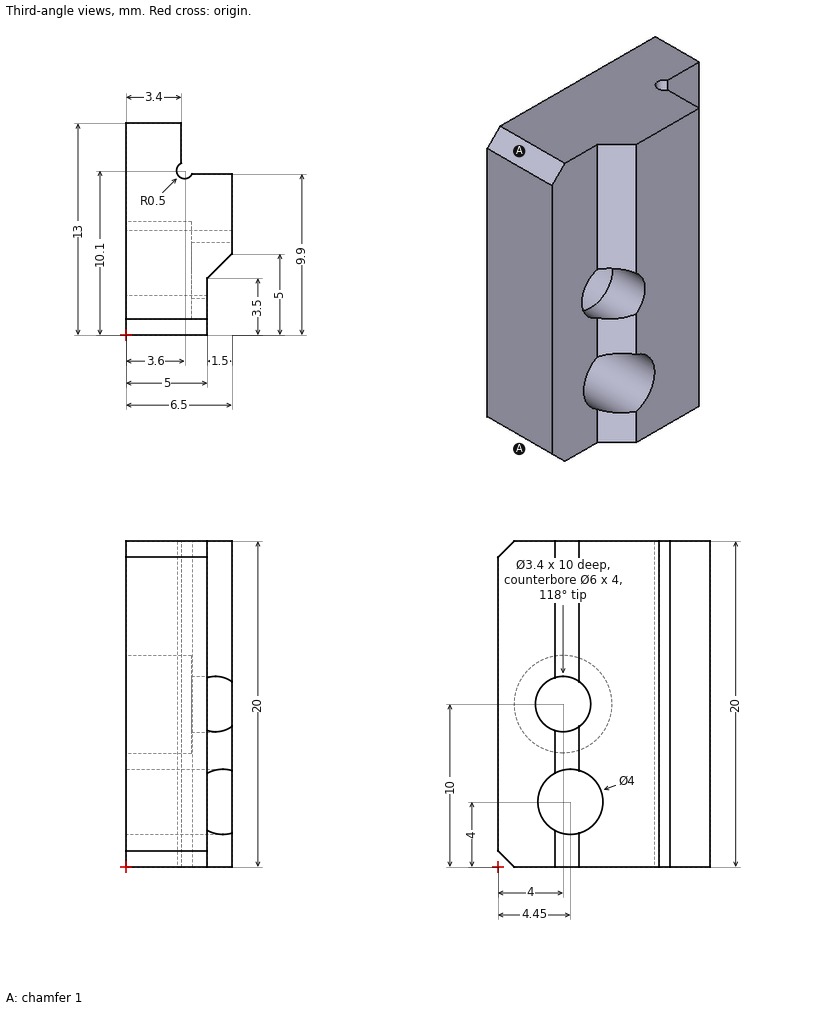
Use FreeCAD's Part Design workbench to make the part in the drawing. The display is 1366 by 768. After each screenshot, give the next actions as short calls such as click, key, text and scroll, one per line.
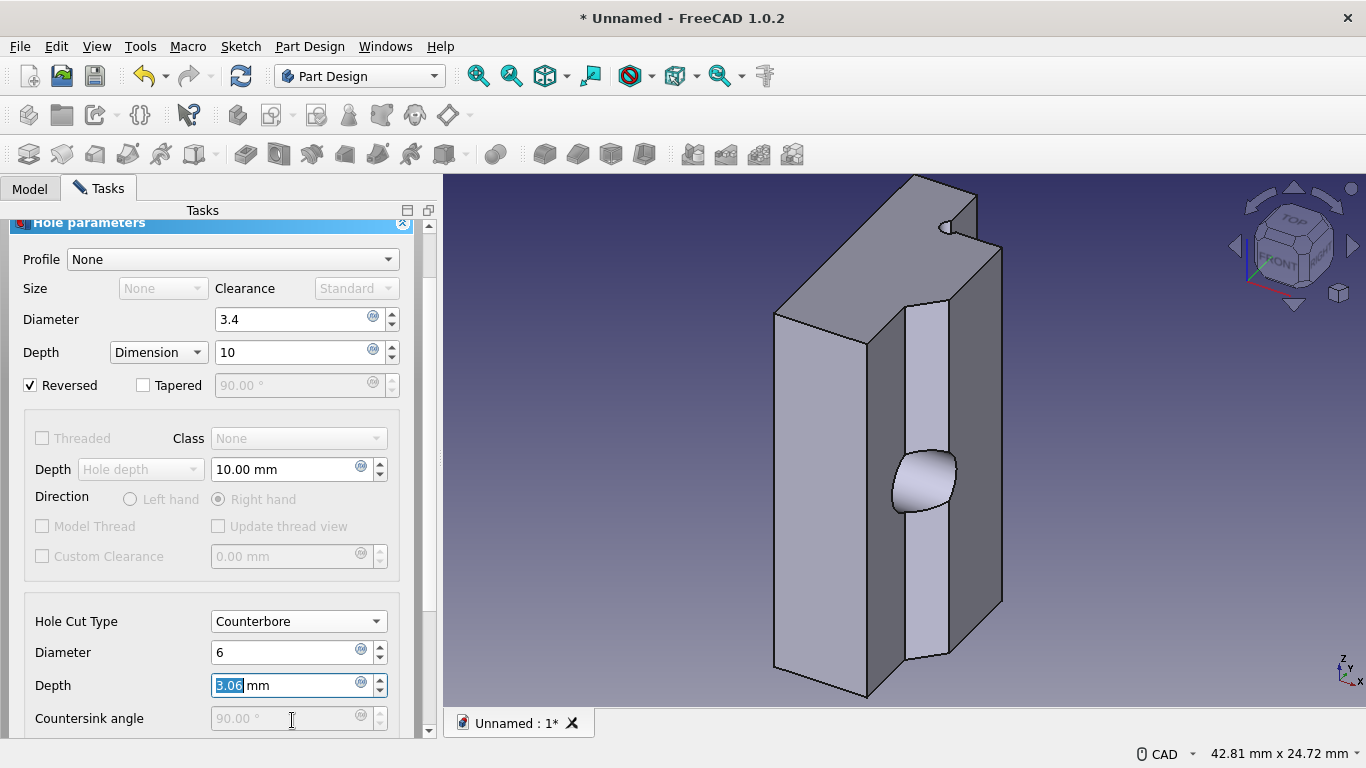
text(4)
key(Tab)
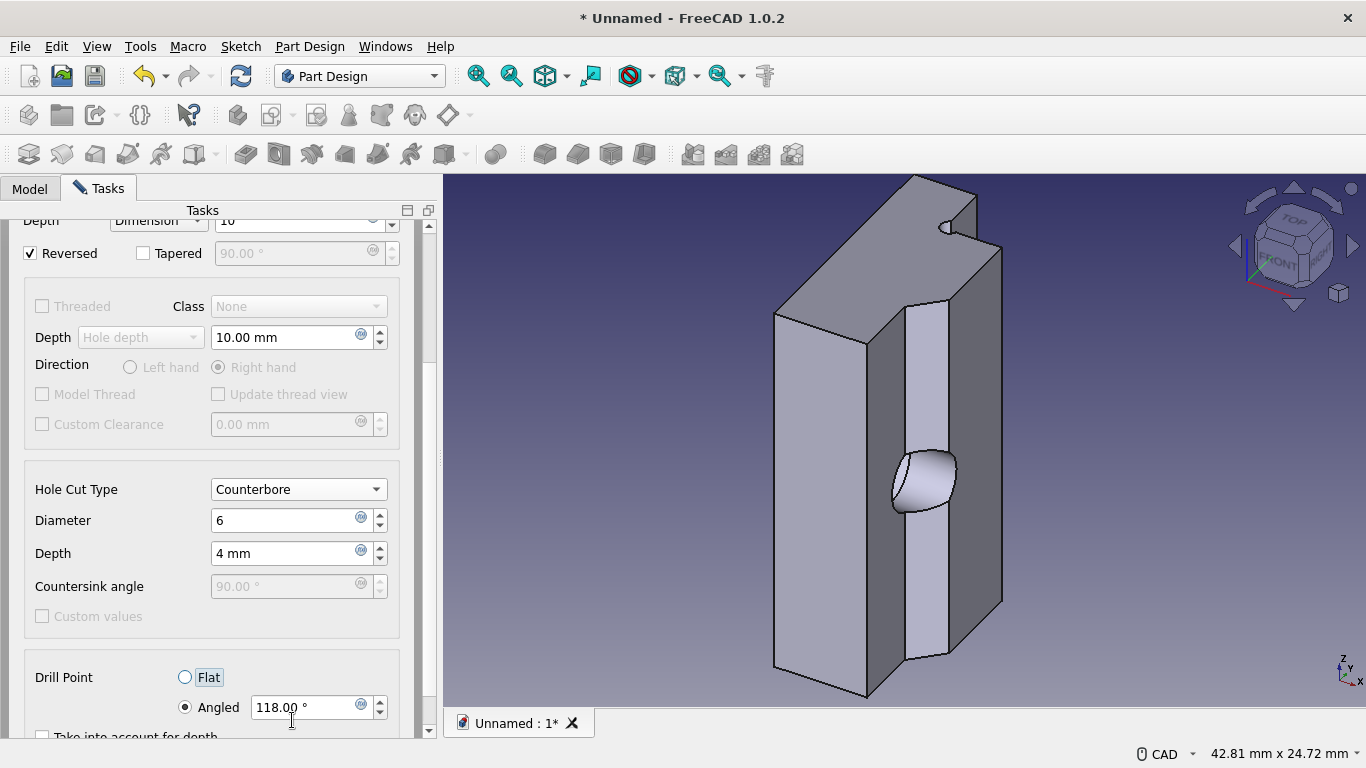
scroll(429, 479, up, 5)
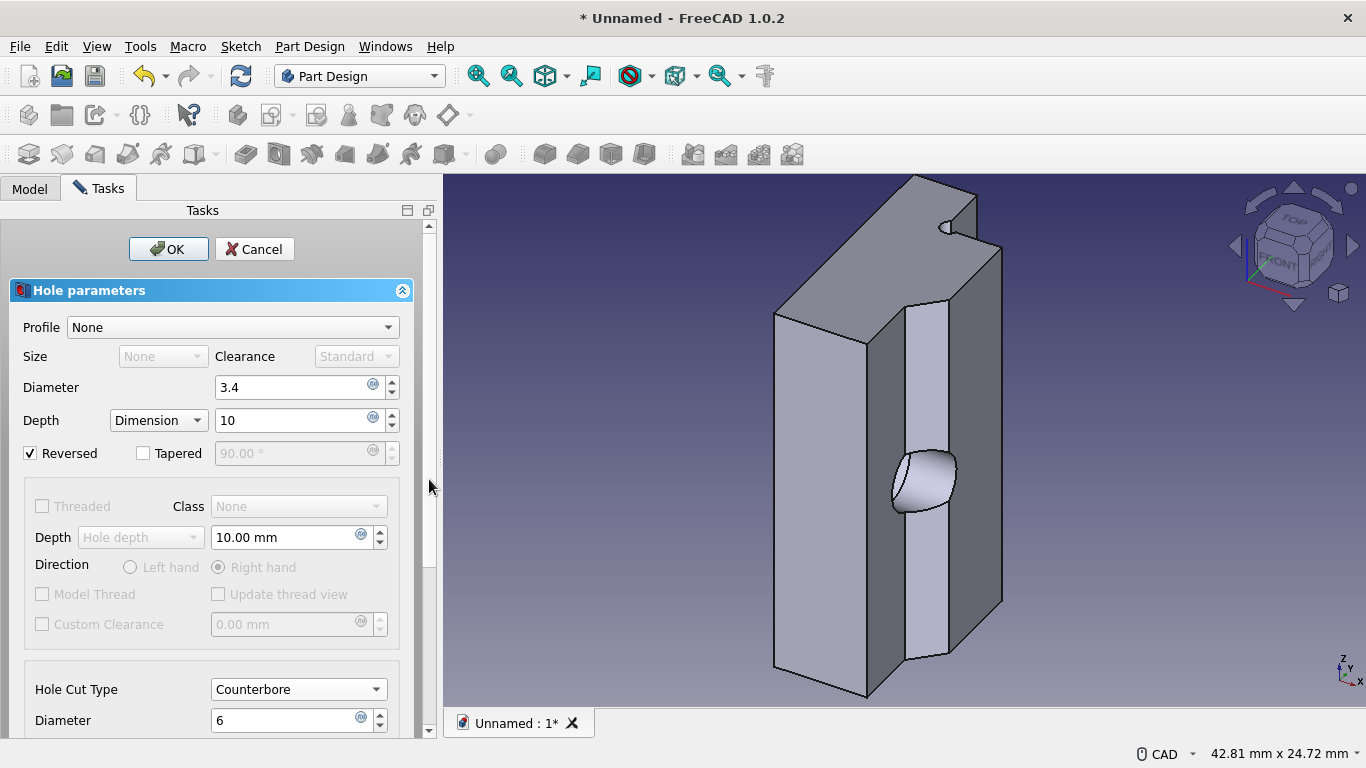
click(169, 249)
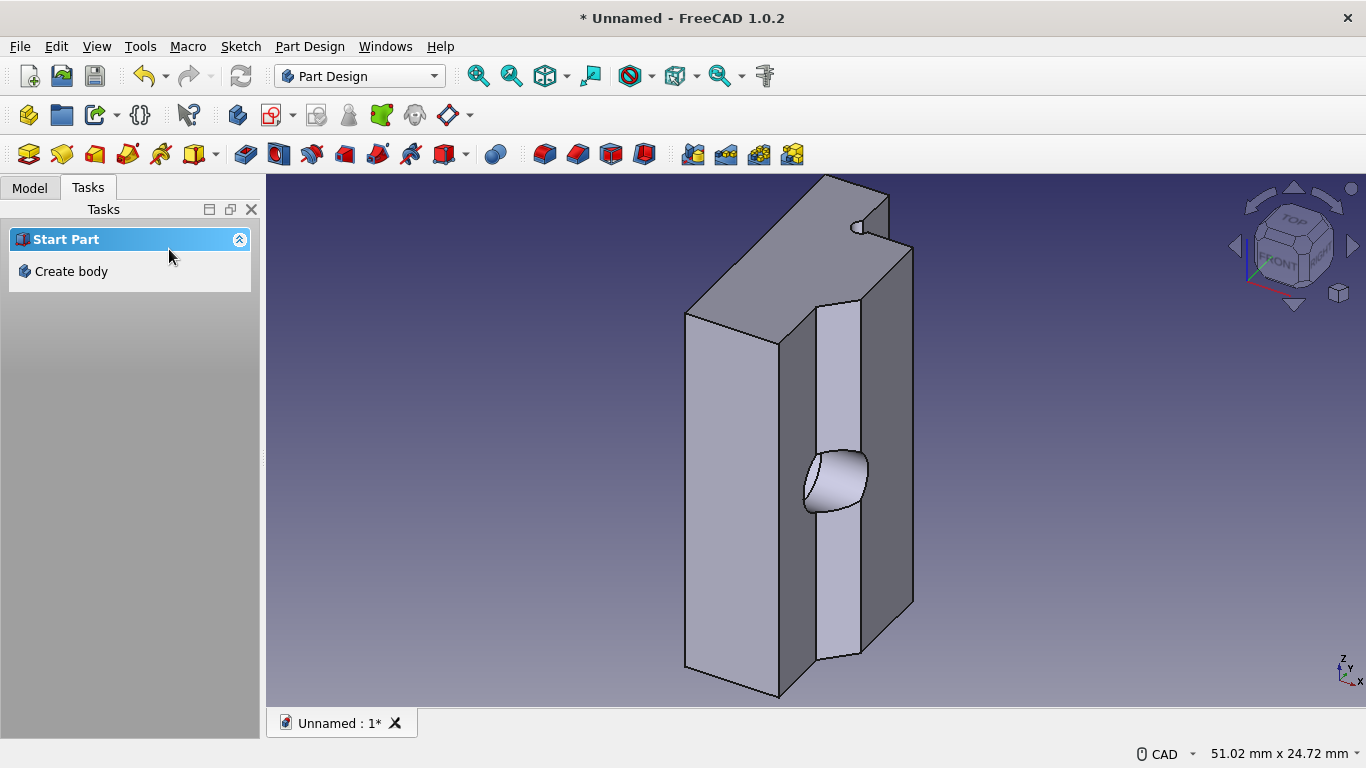
click(479, 76)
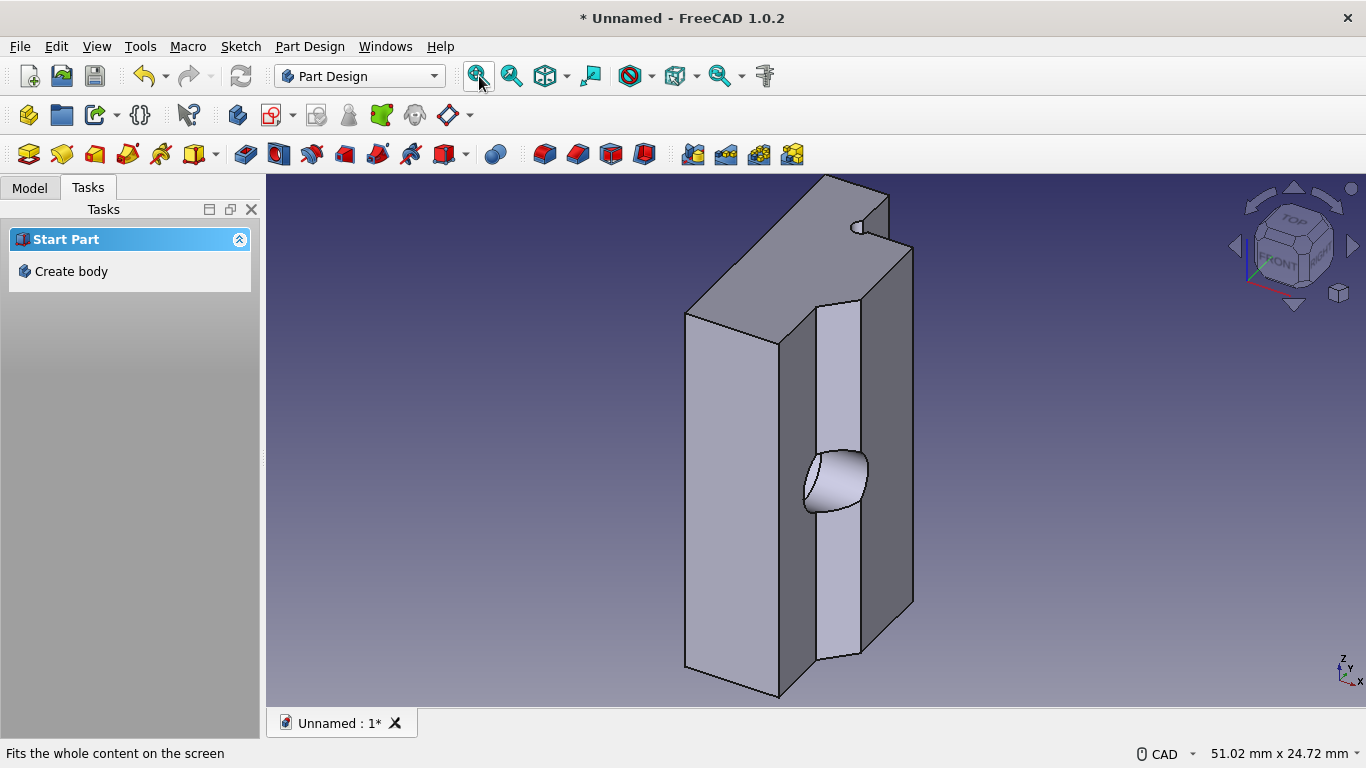
click(732, 328)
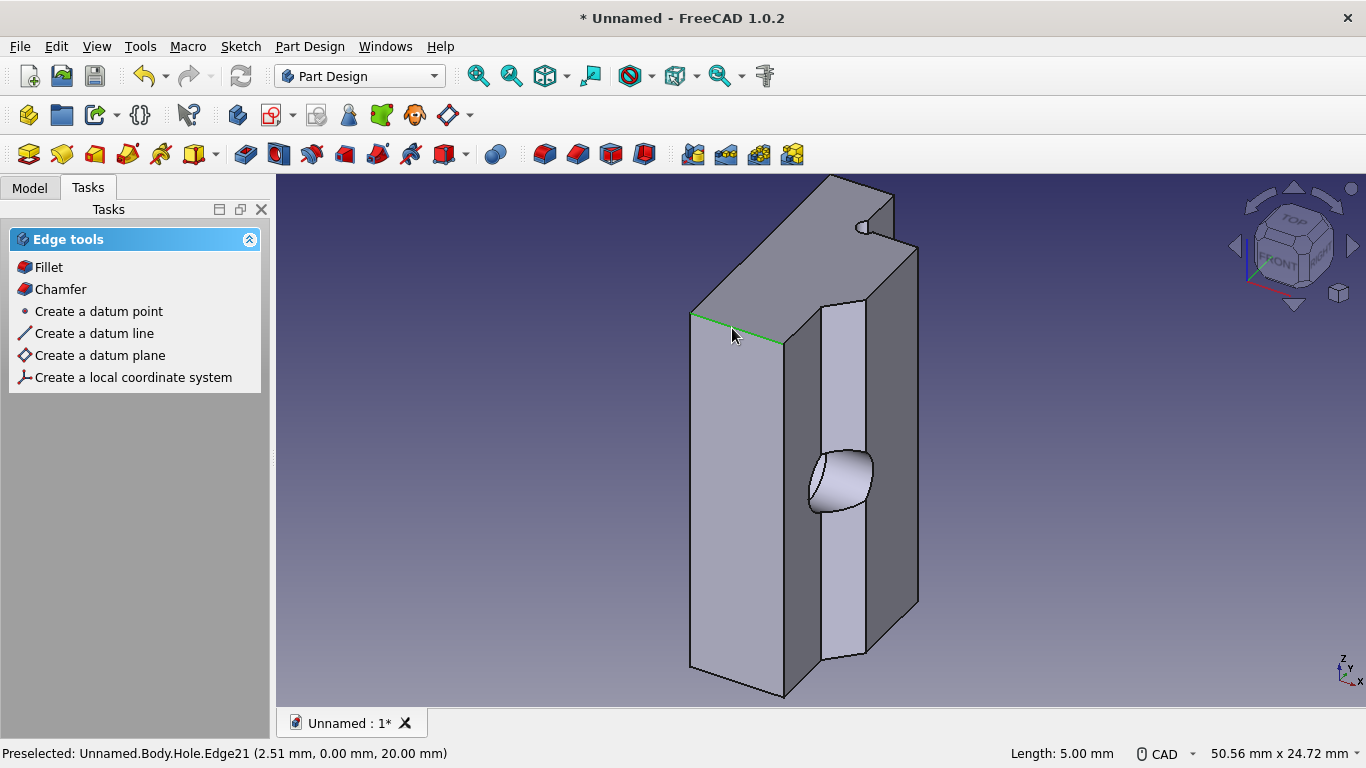
key(0)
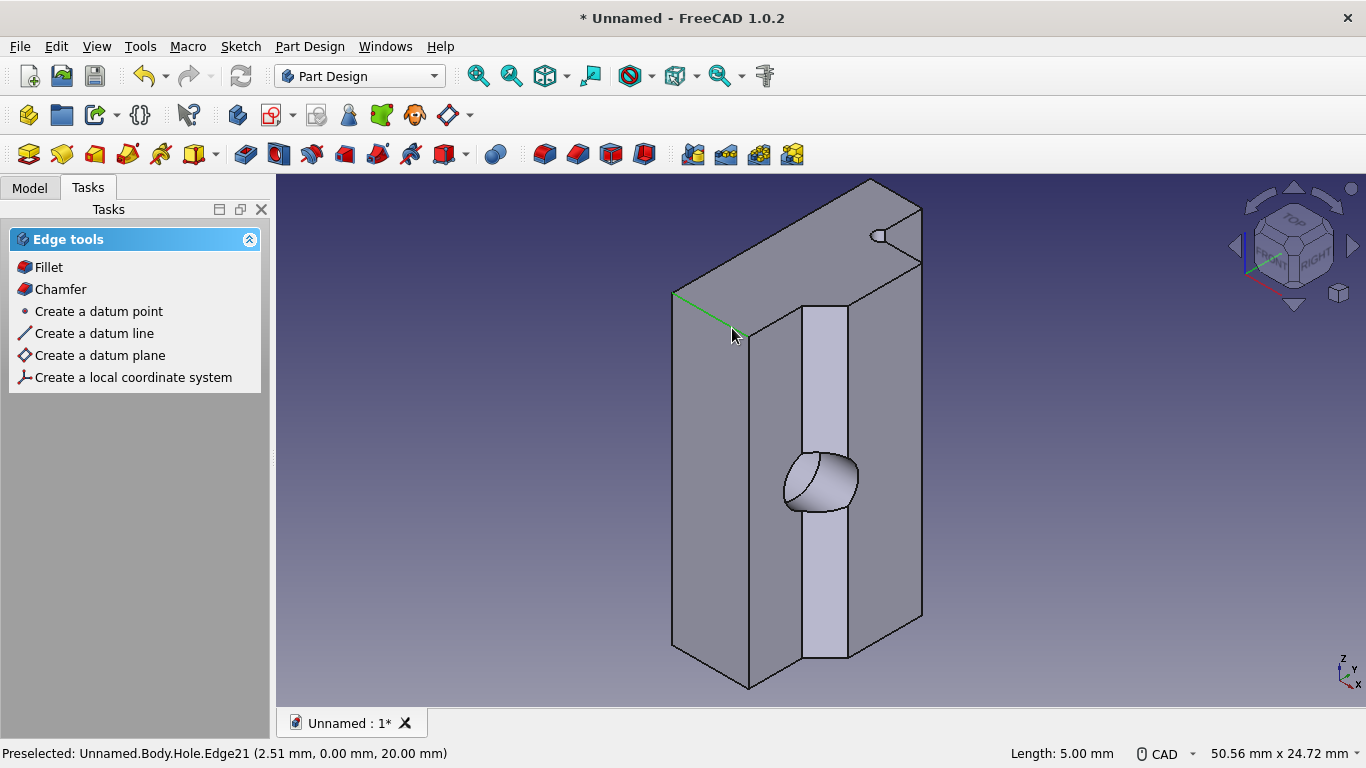
key(2)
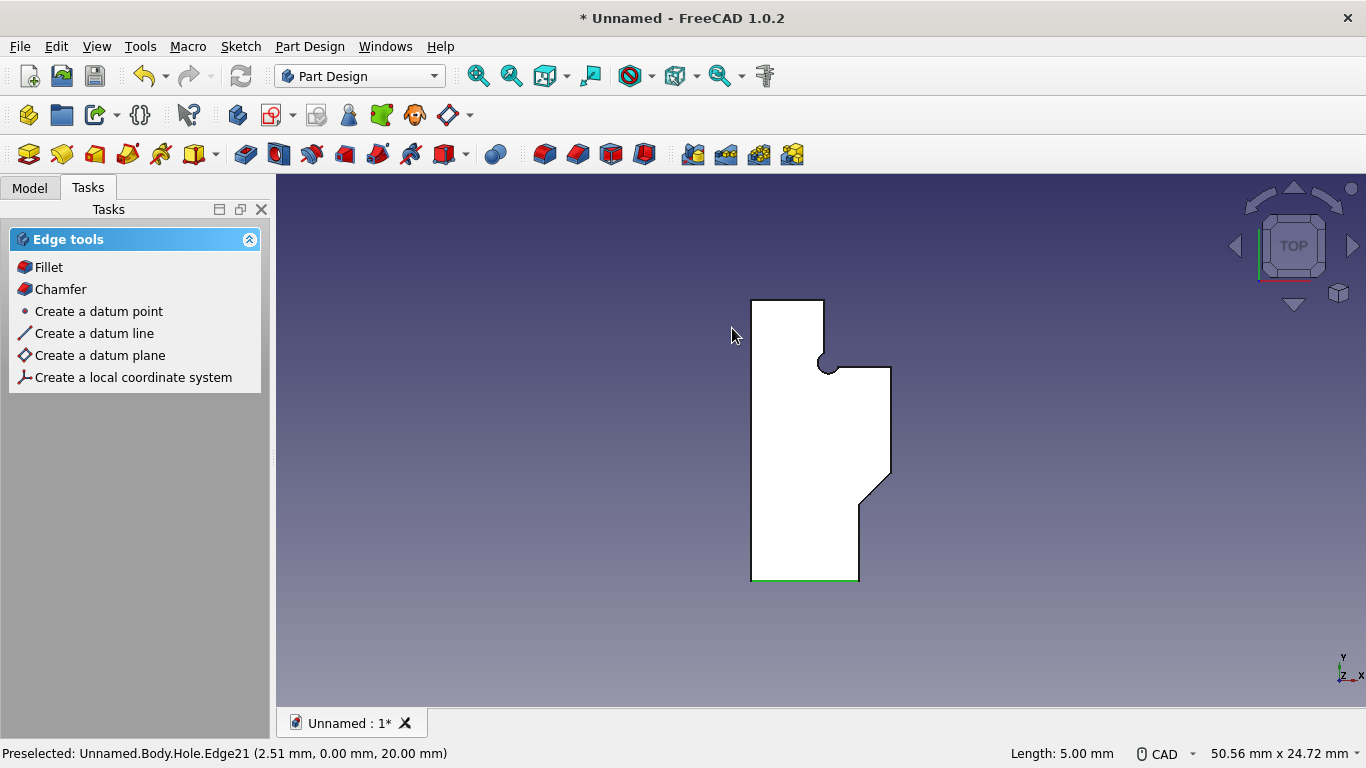
key(1)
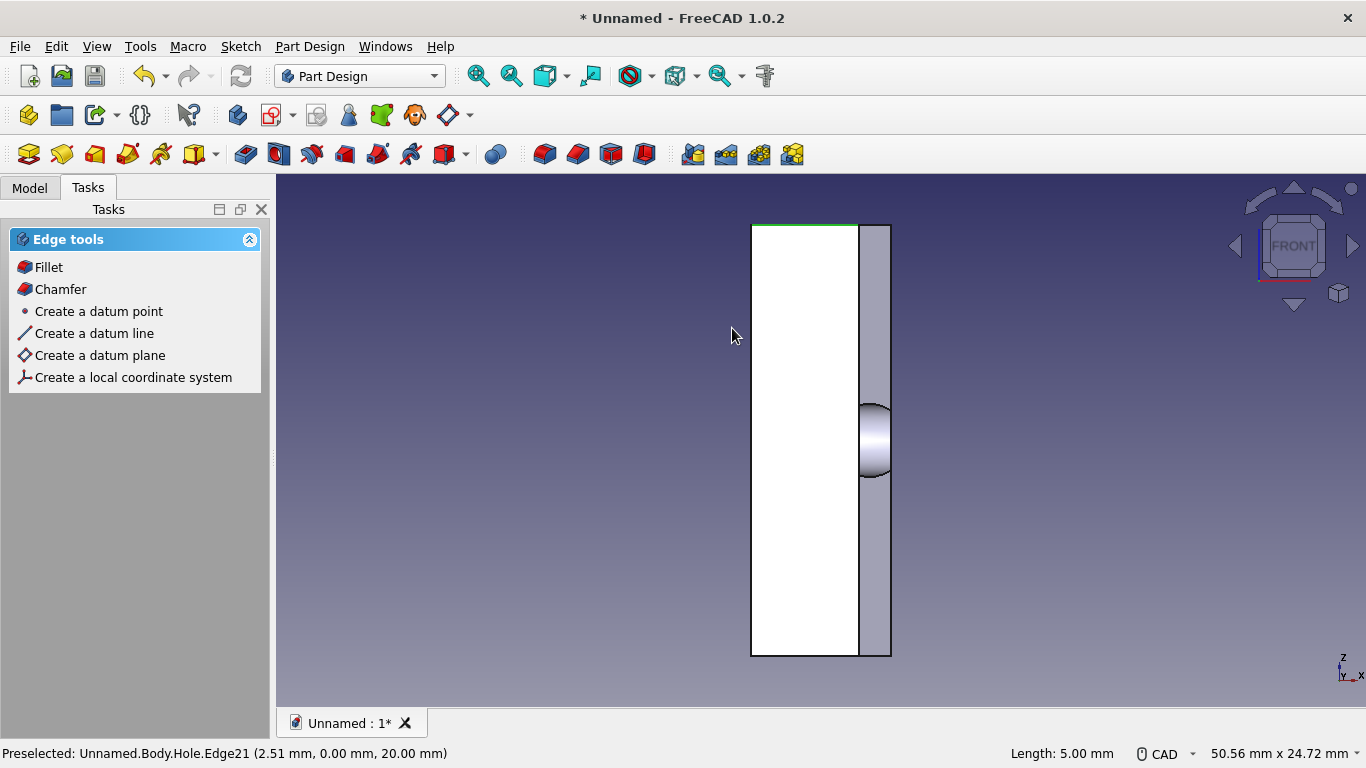
click(805, 655, ctrl)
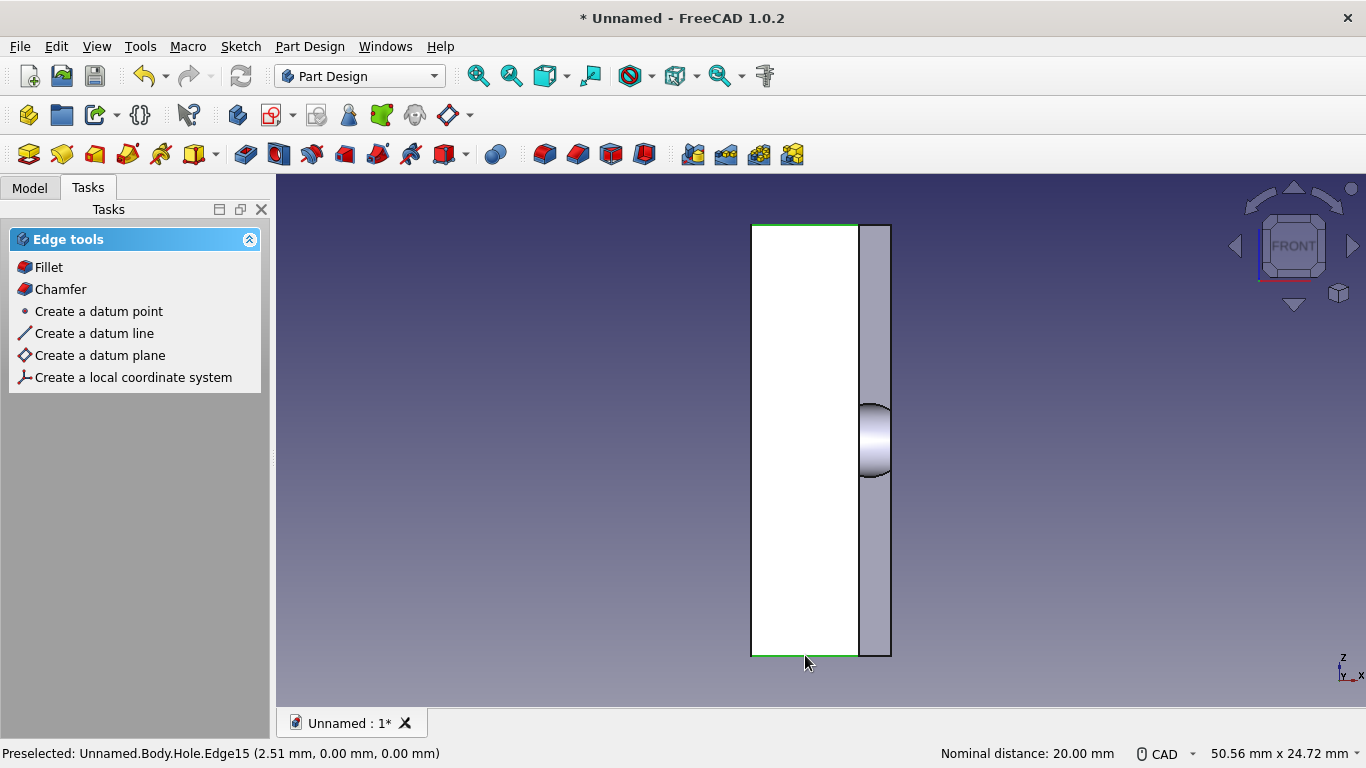
click(578, 154)